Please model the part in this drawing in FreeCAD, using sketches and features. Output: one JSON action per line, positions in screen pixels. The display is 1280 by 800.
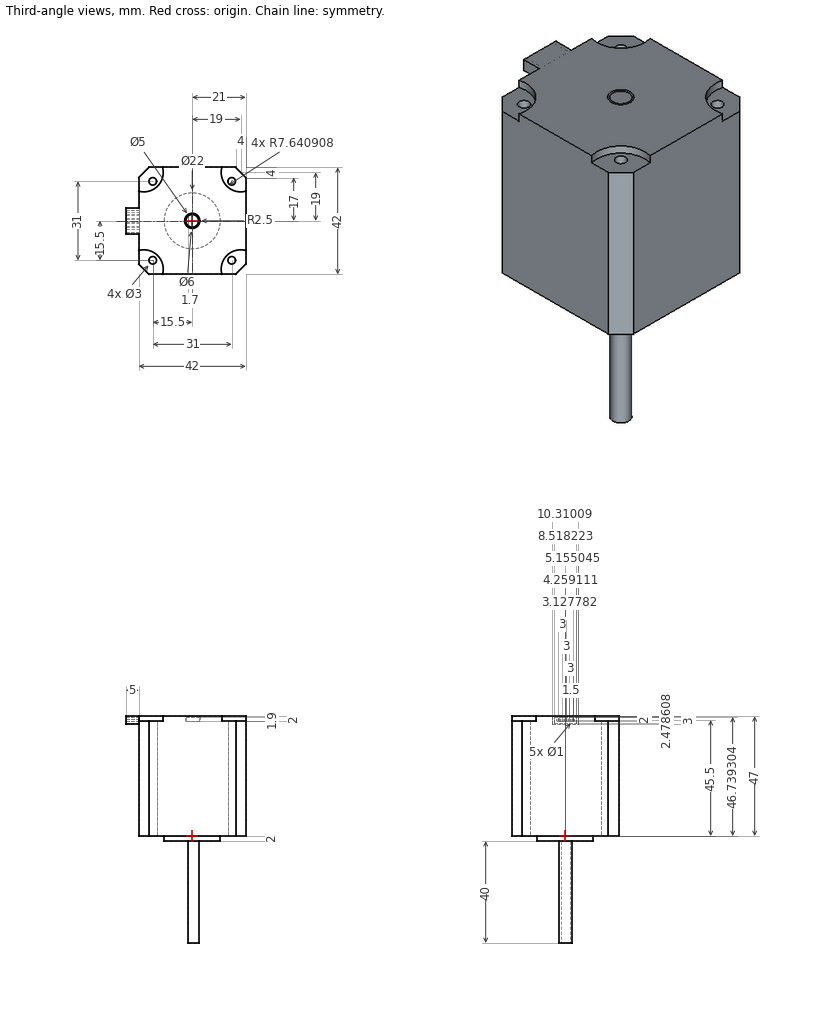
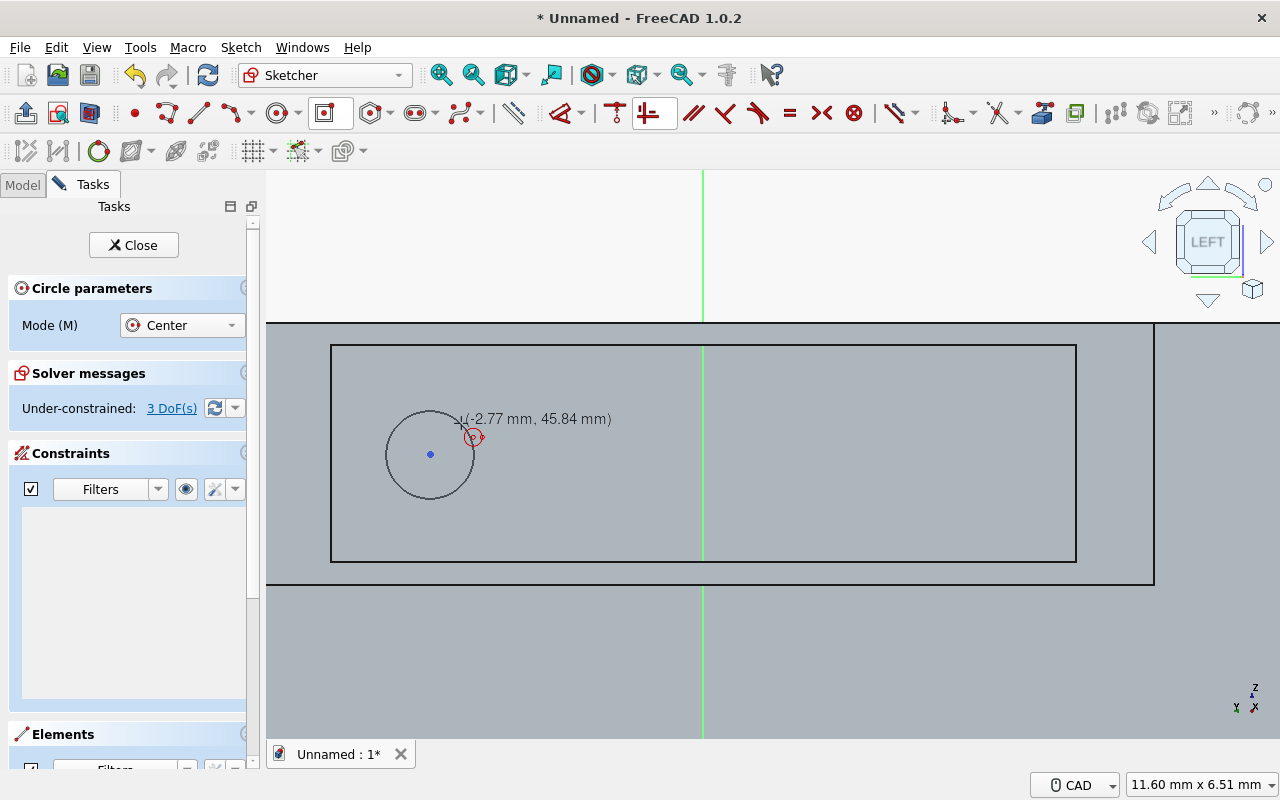
{"action": "left_click", "coordinate": [561, 454]}
{"action": "left_click", "coordinate": [592, 423]}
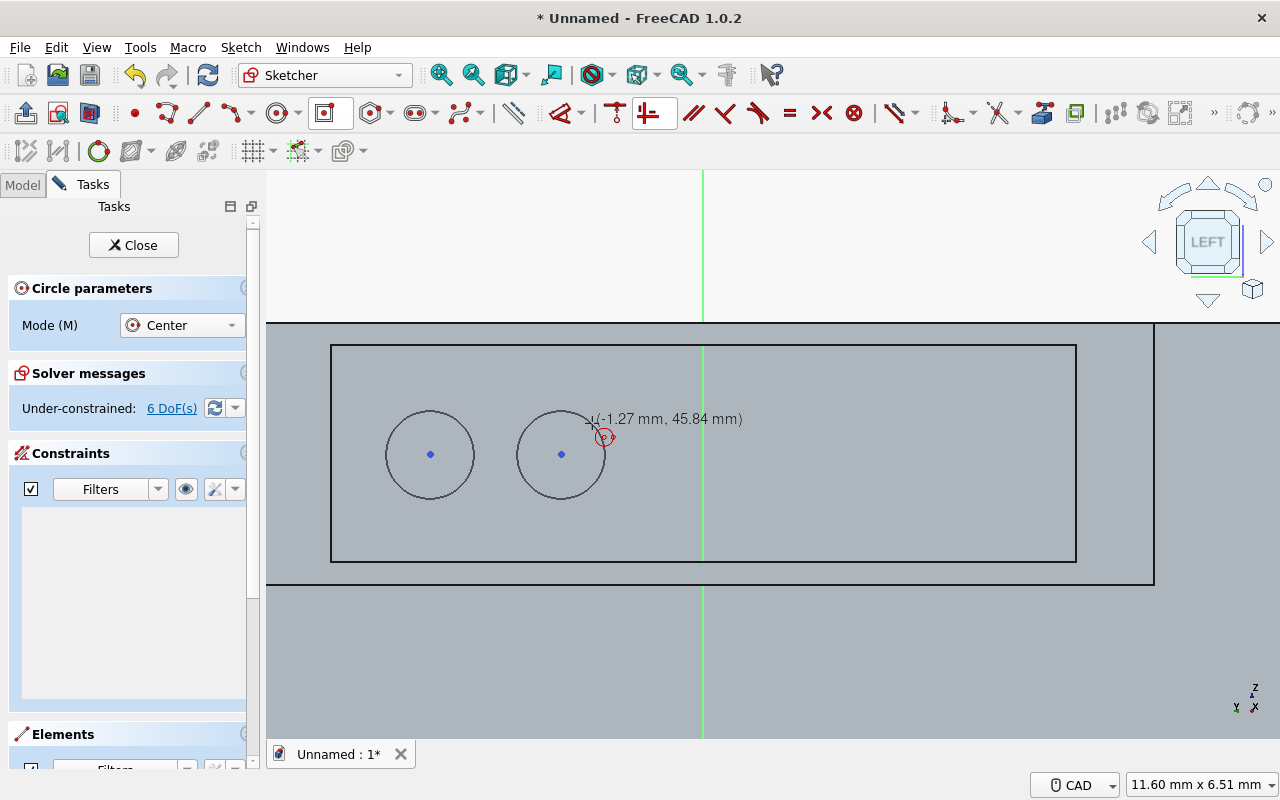
{"action": "scroll", "coordinate": [692, 454], "scroll_direction": "up", "scroll_amount": 2}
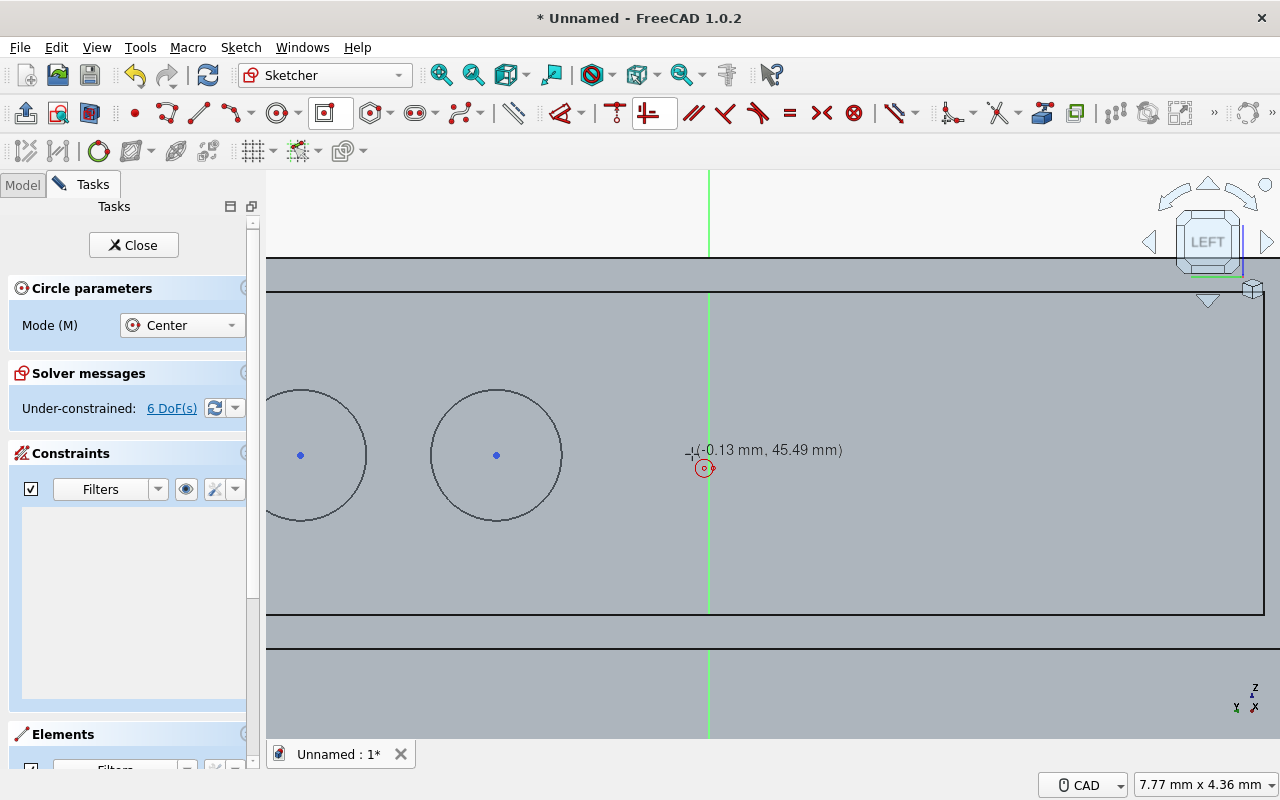
{"action": "left_click", "coordinate": [692, 454]}
{"action": "left_click", "coordinate": [738, 407]}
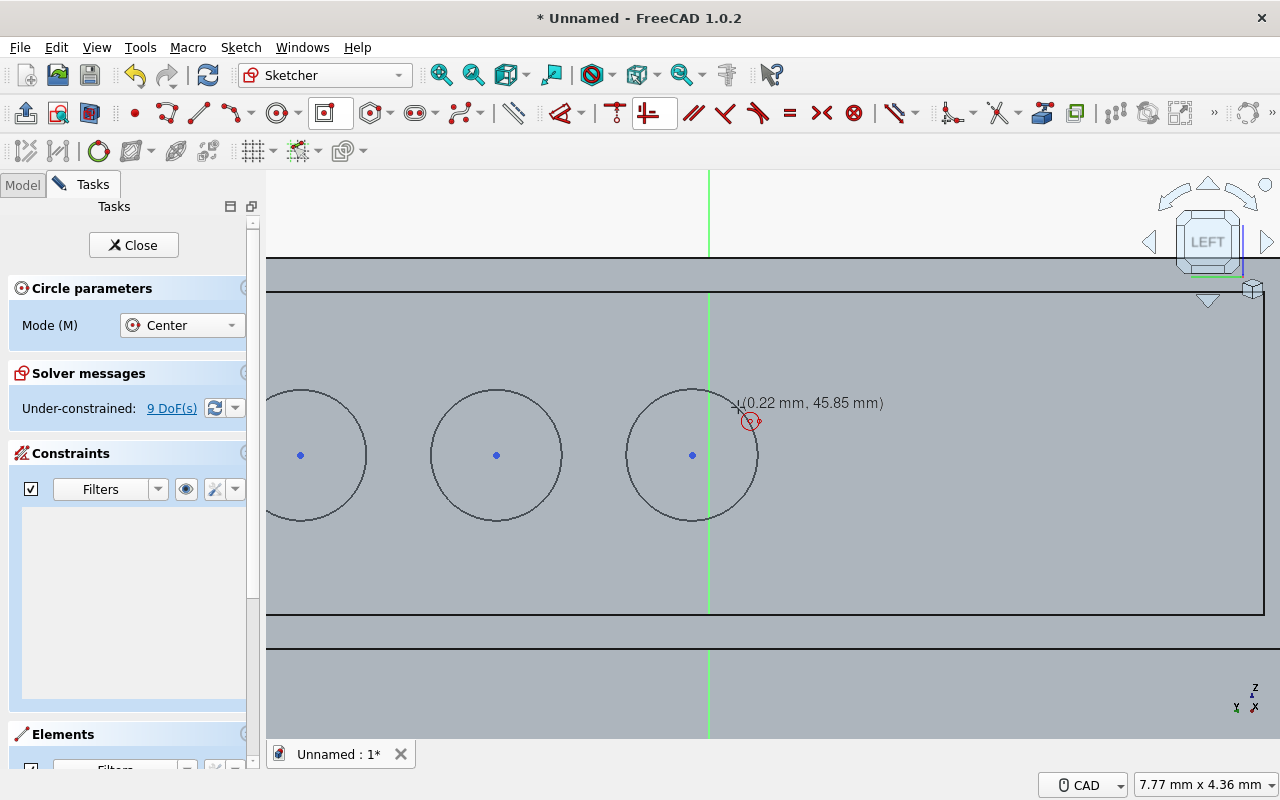
{"action": "left_click", "coordinate": [888, 454]}
{"action": "left_click", "coordinate": [934, 407]}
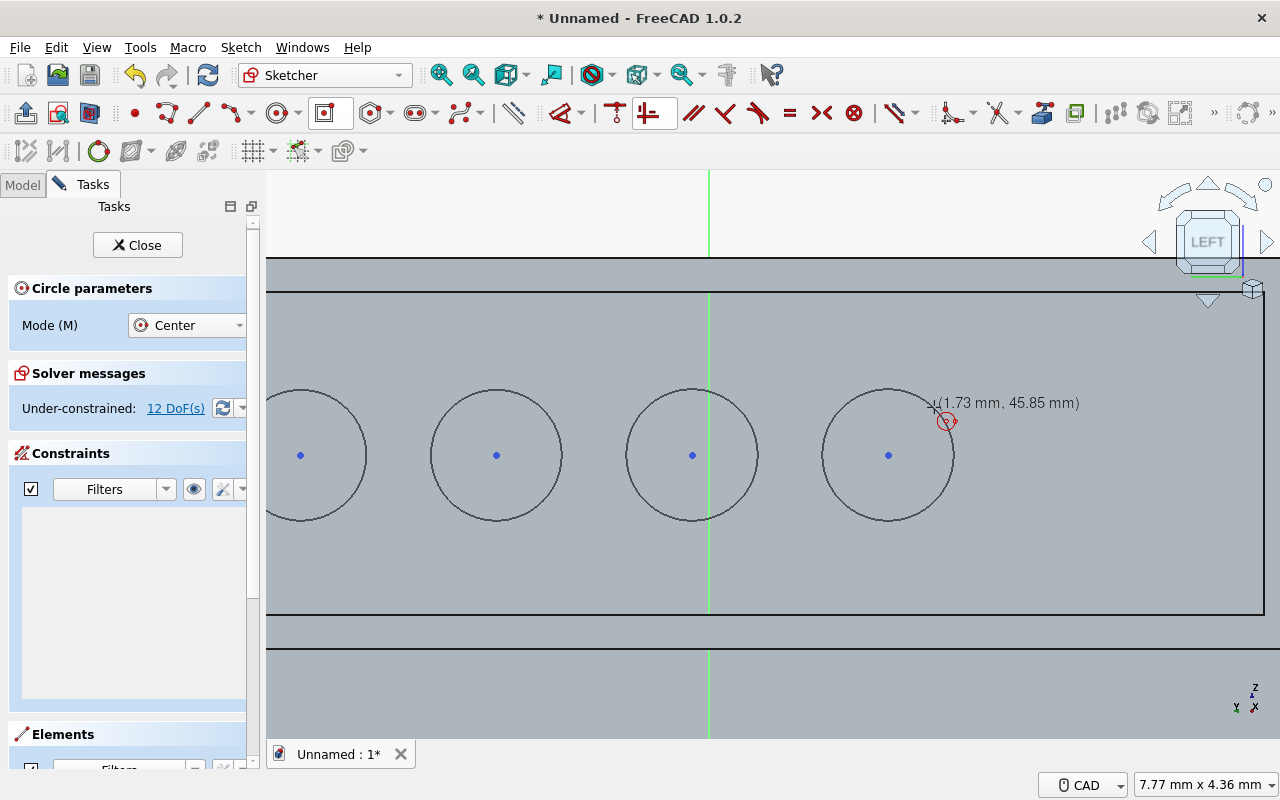
{"action": "left_click", "coordinate": [1084, 454]}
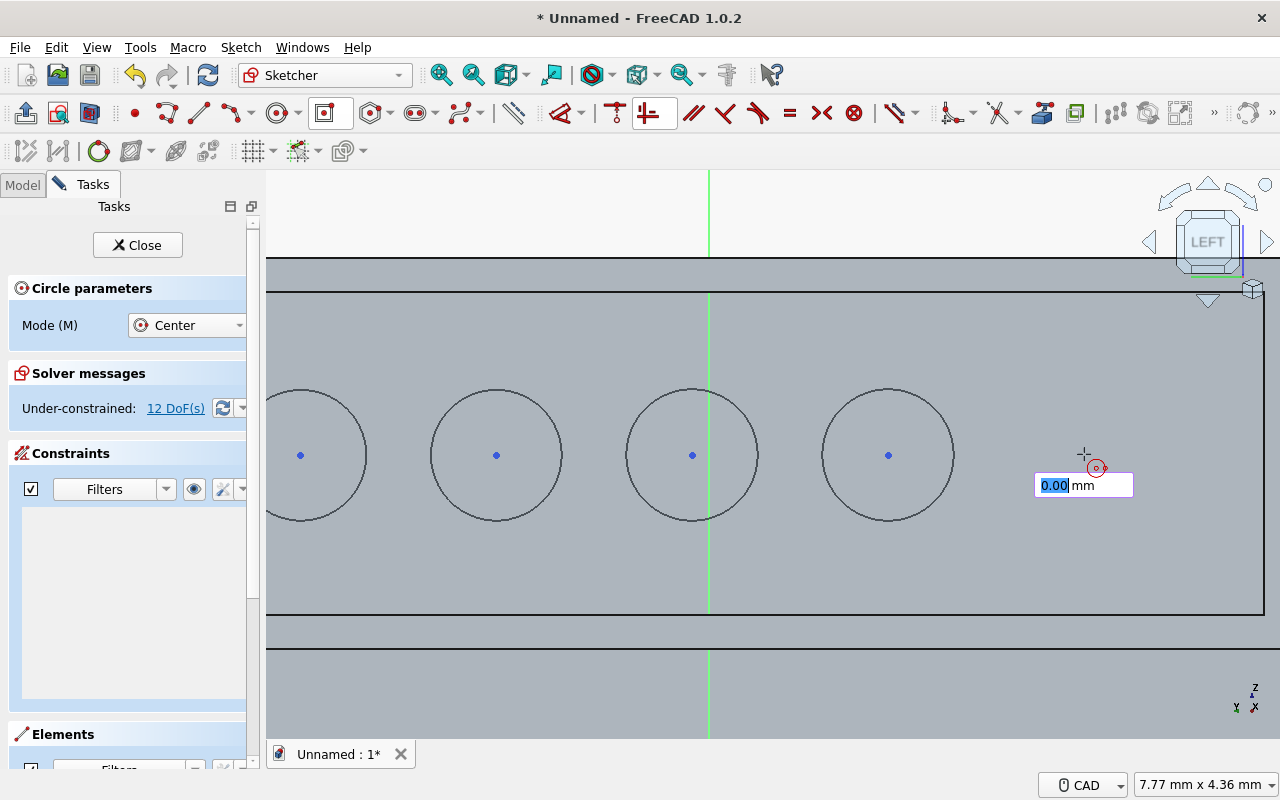
{"action": "scroll", "coordinate": [730, 456], "scroll_direction": "down", "scroll_amount": 2}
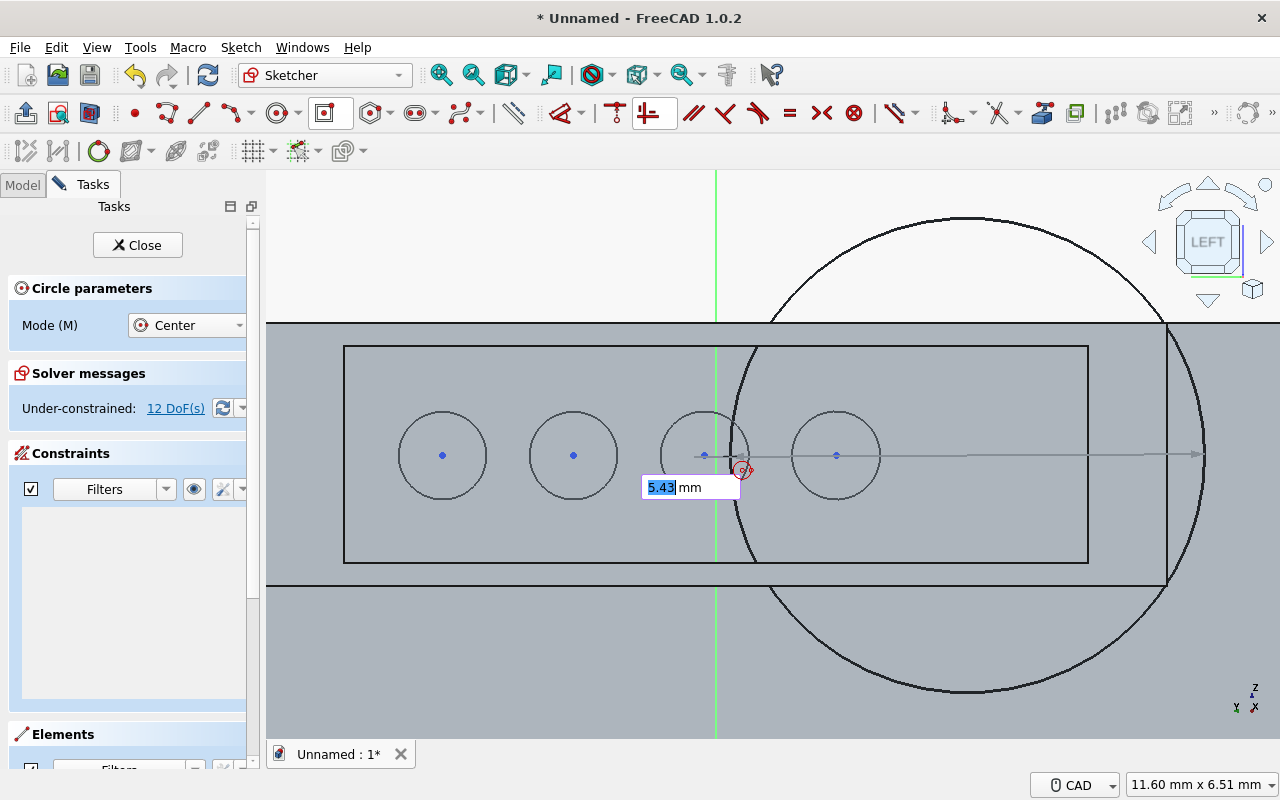
{"action": "left_click", "coordinate": [998, 424]}
{"action": "key", "text": "Escape"}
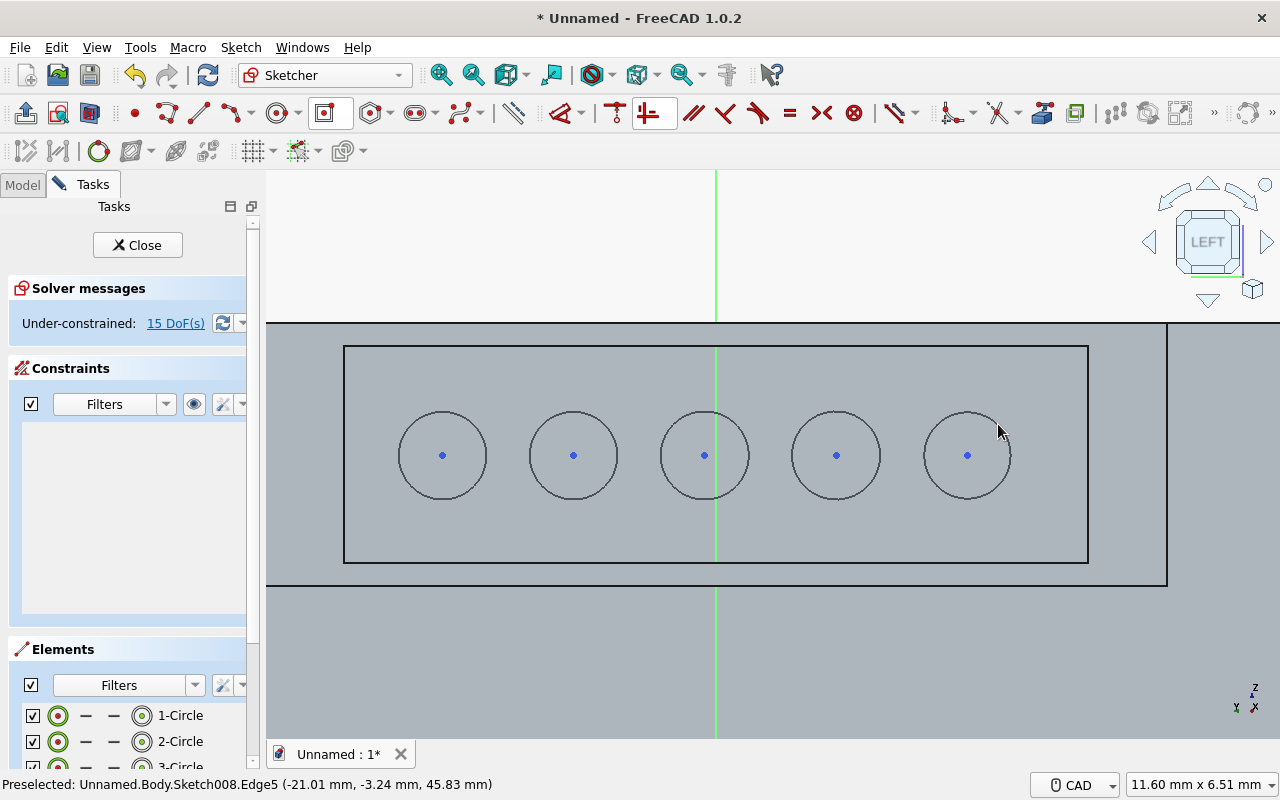
{"action": "left_click", "coordinate": [473, 425]}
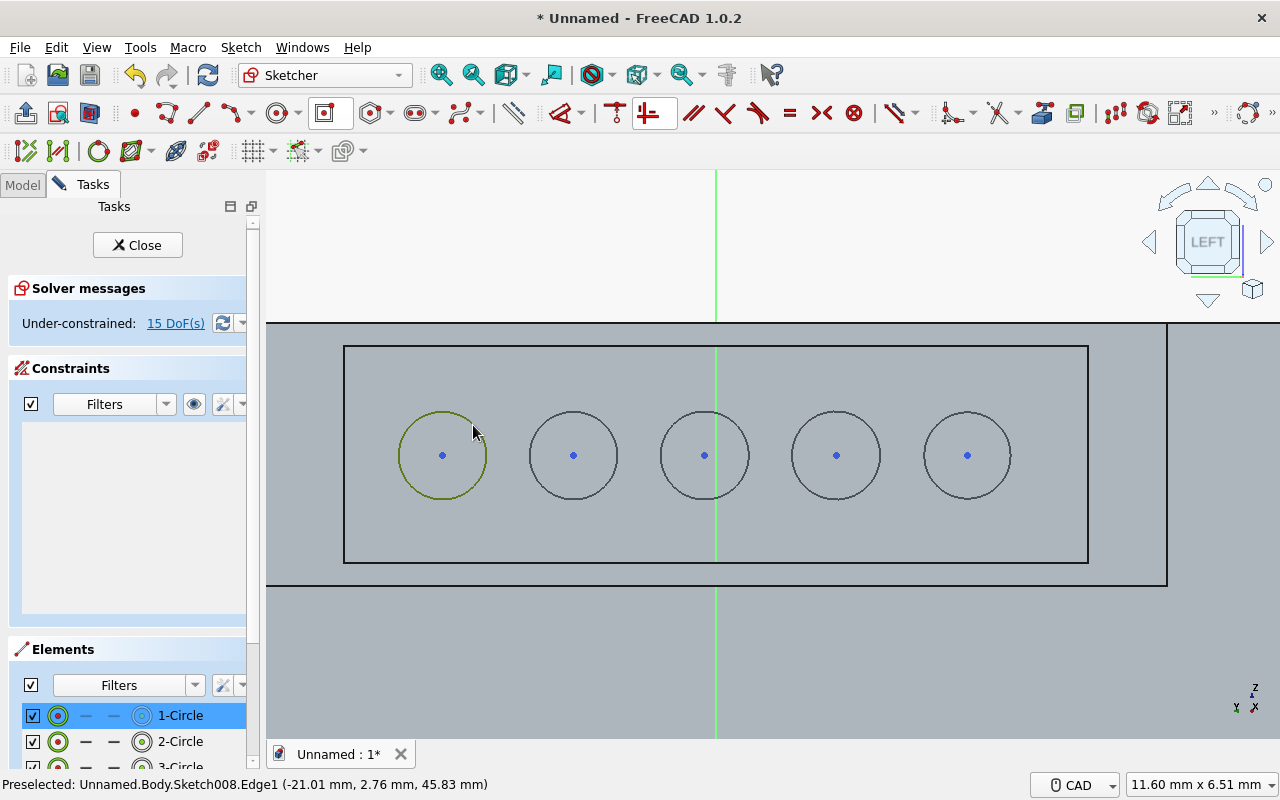
{"action": "left_click", "coordinate": [604, 425]}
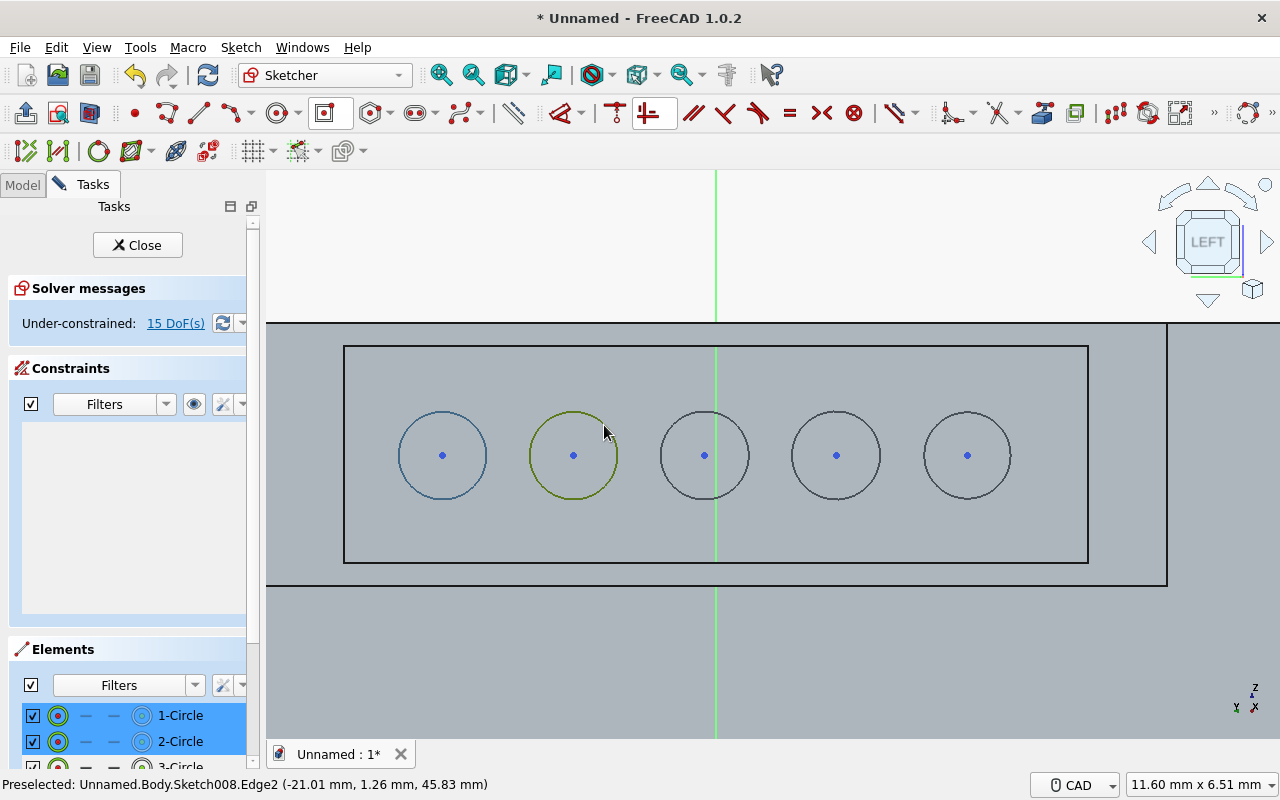
{"action": "left_click", "coordinate": [736, 424]}